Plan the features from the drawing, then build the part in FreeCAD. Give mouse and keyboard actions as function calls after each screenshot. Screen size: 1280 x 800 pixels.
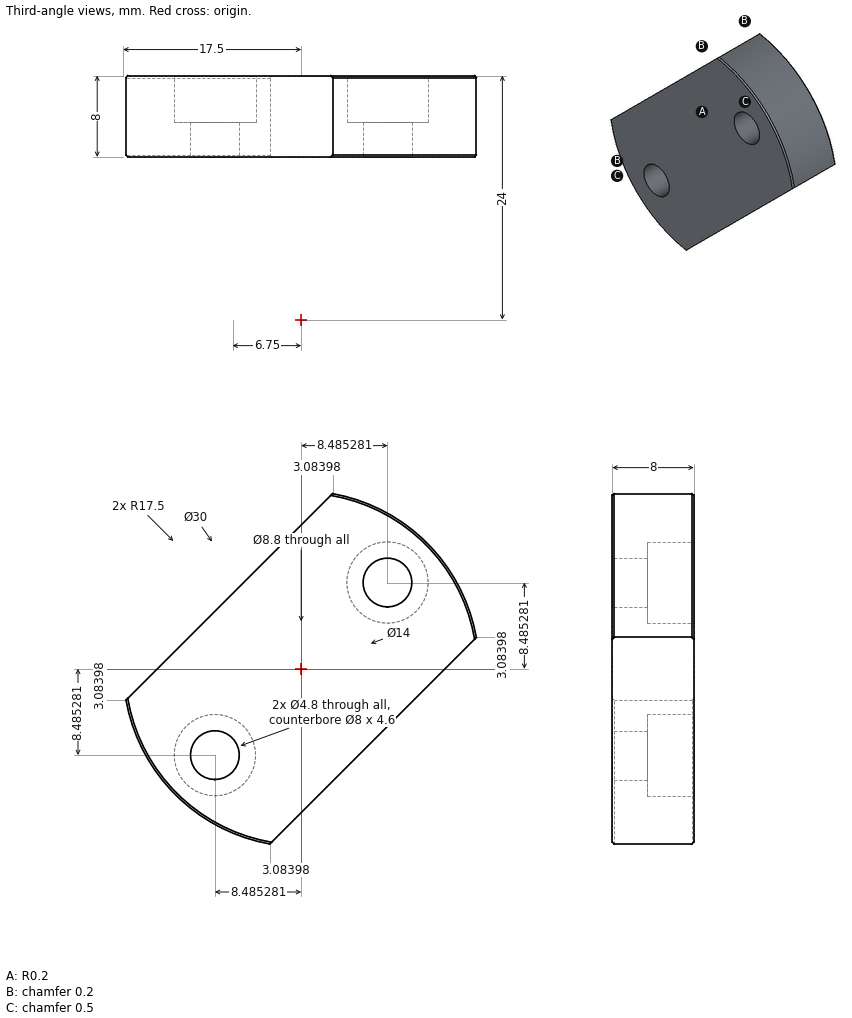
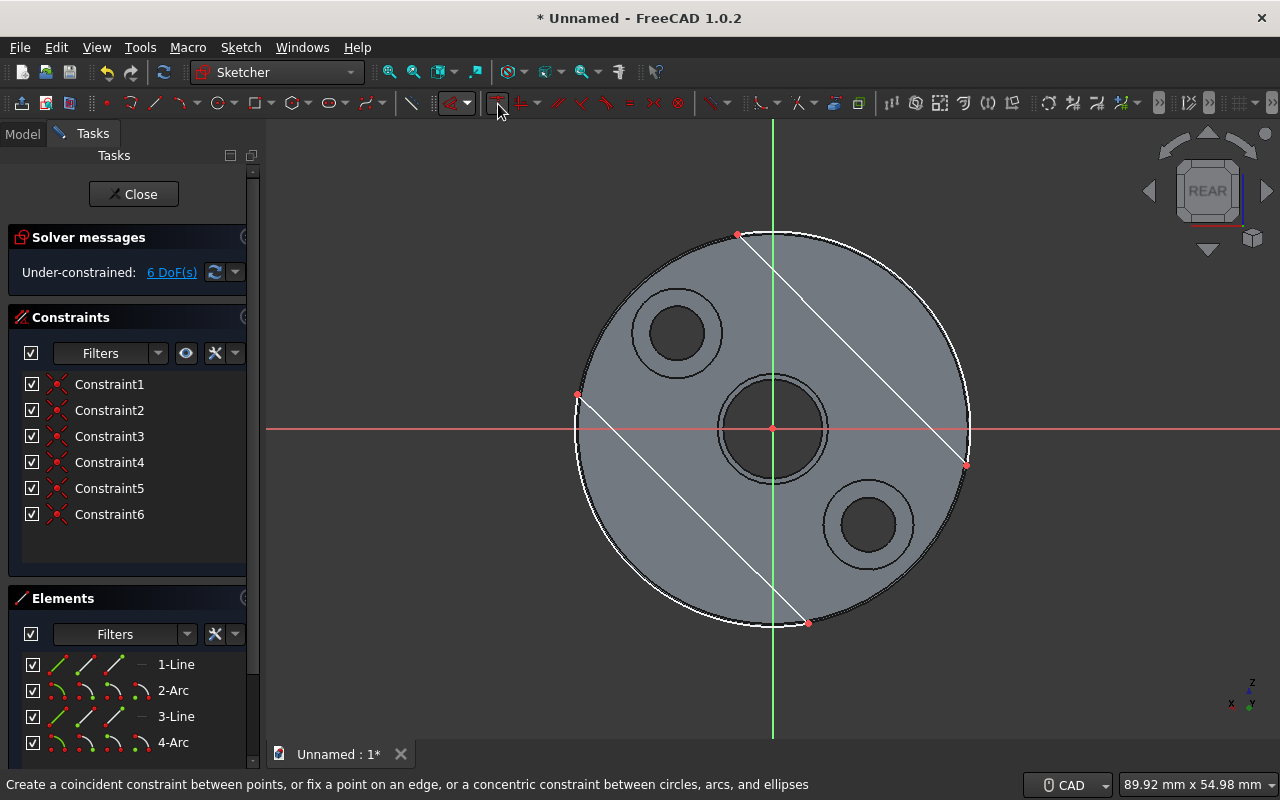
click(955, 353)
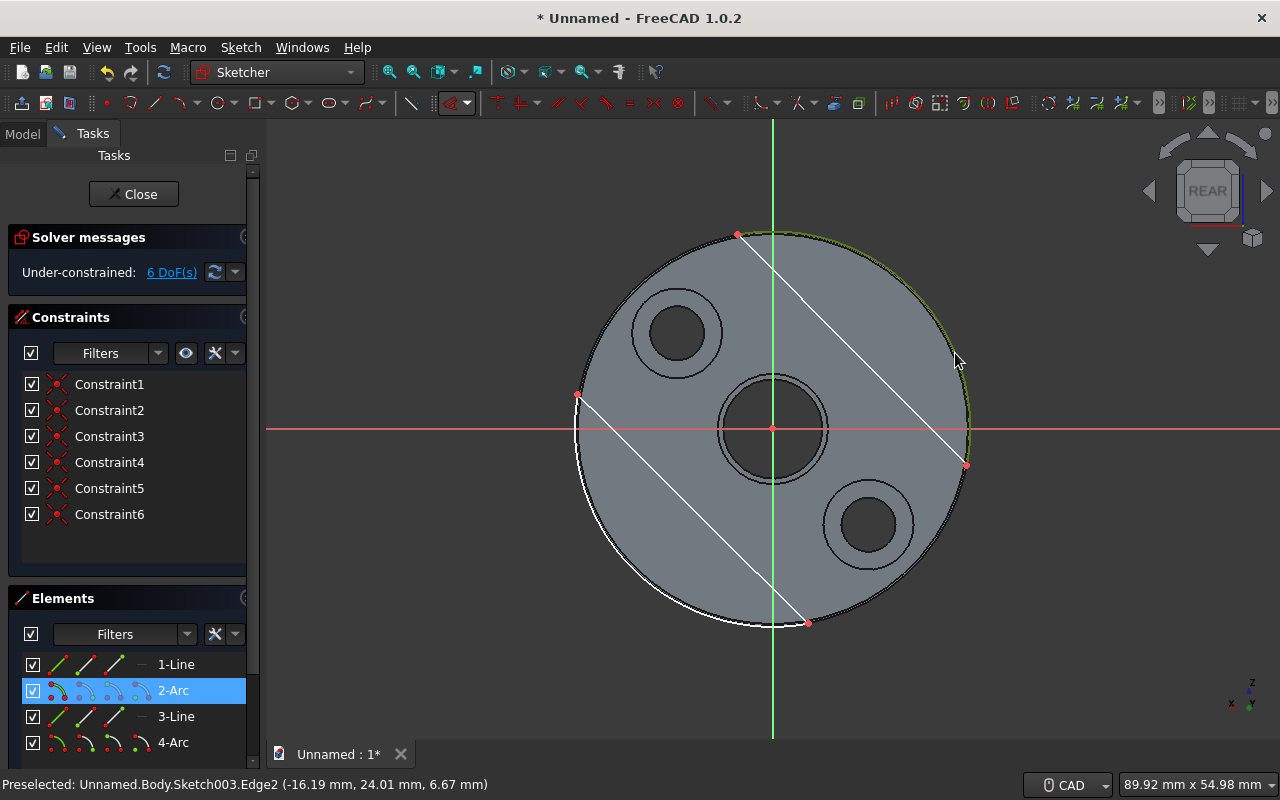
click(591, 507)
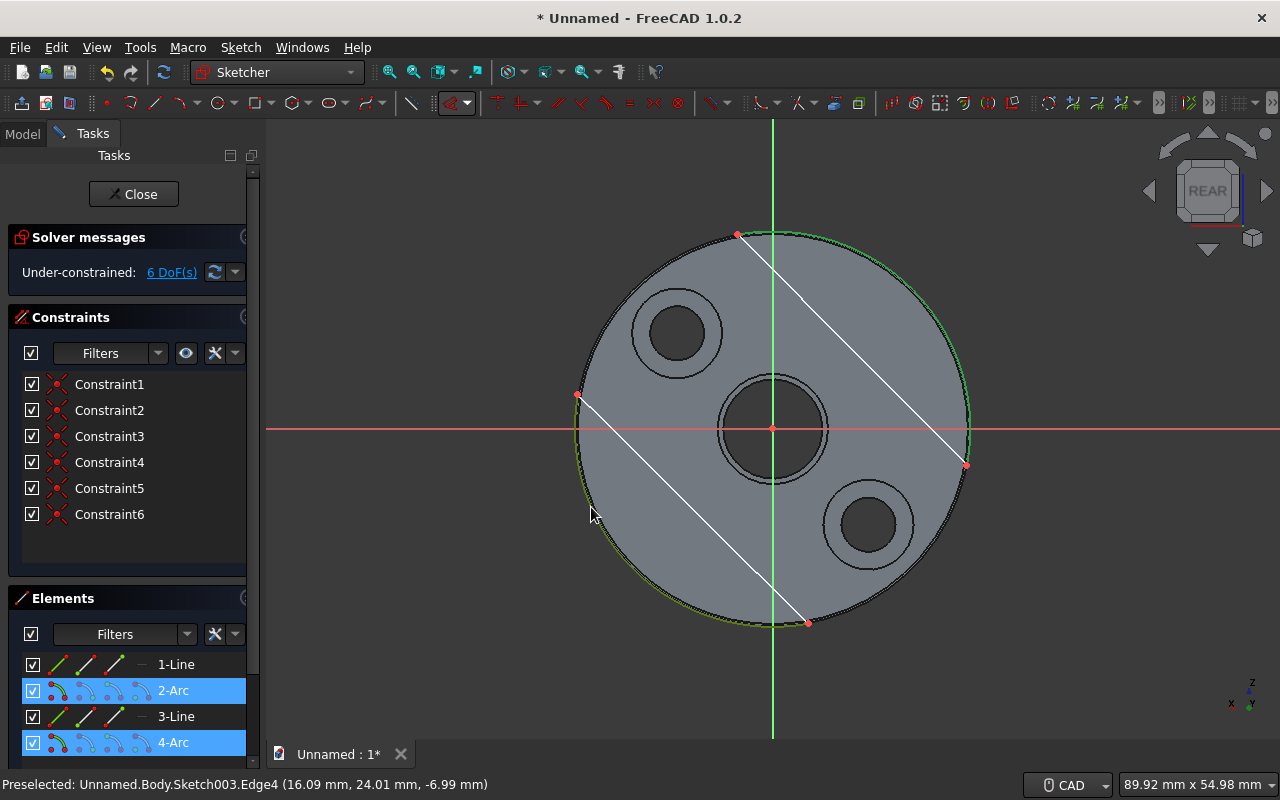
click(630, 104)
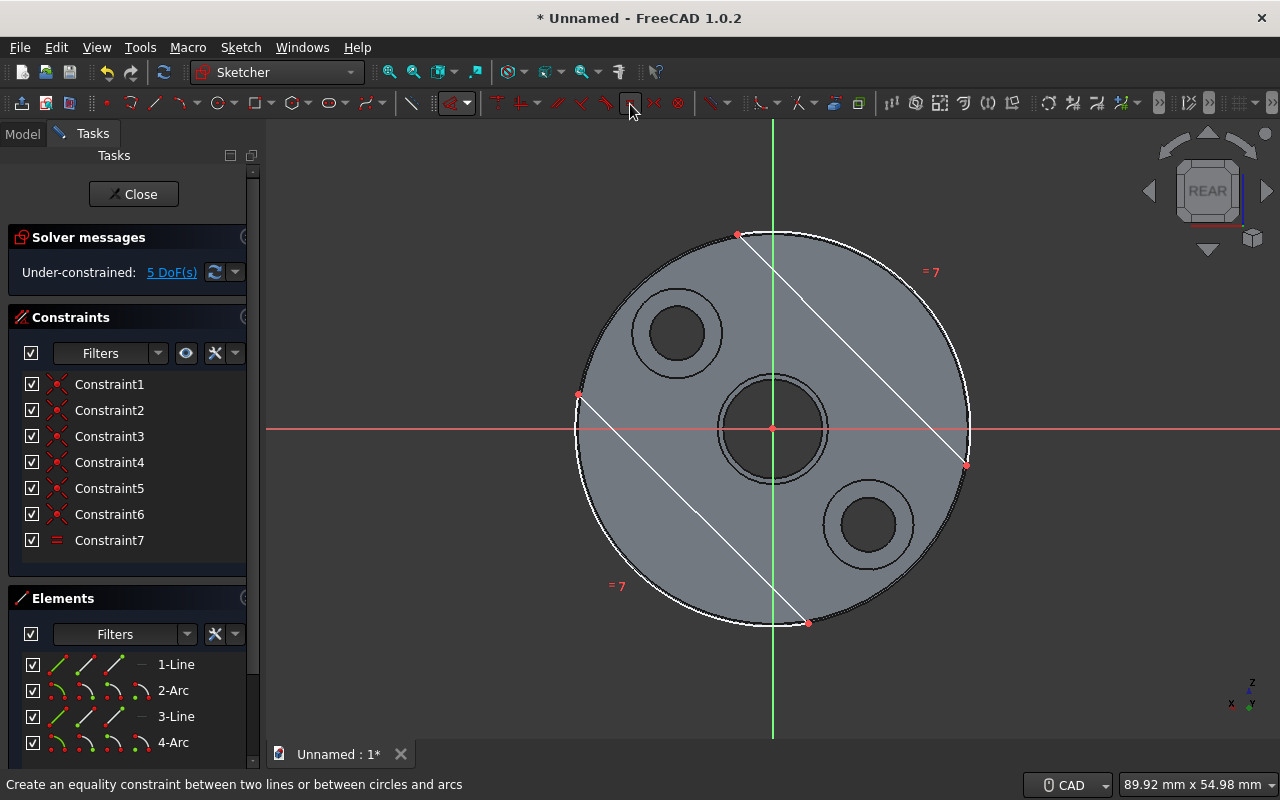
click(955, 353)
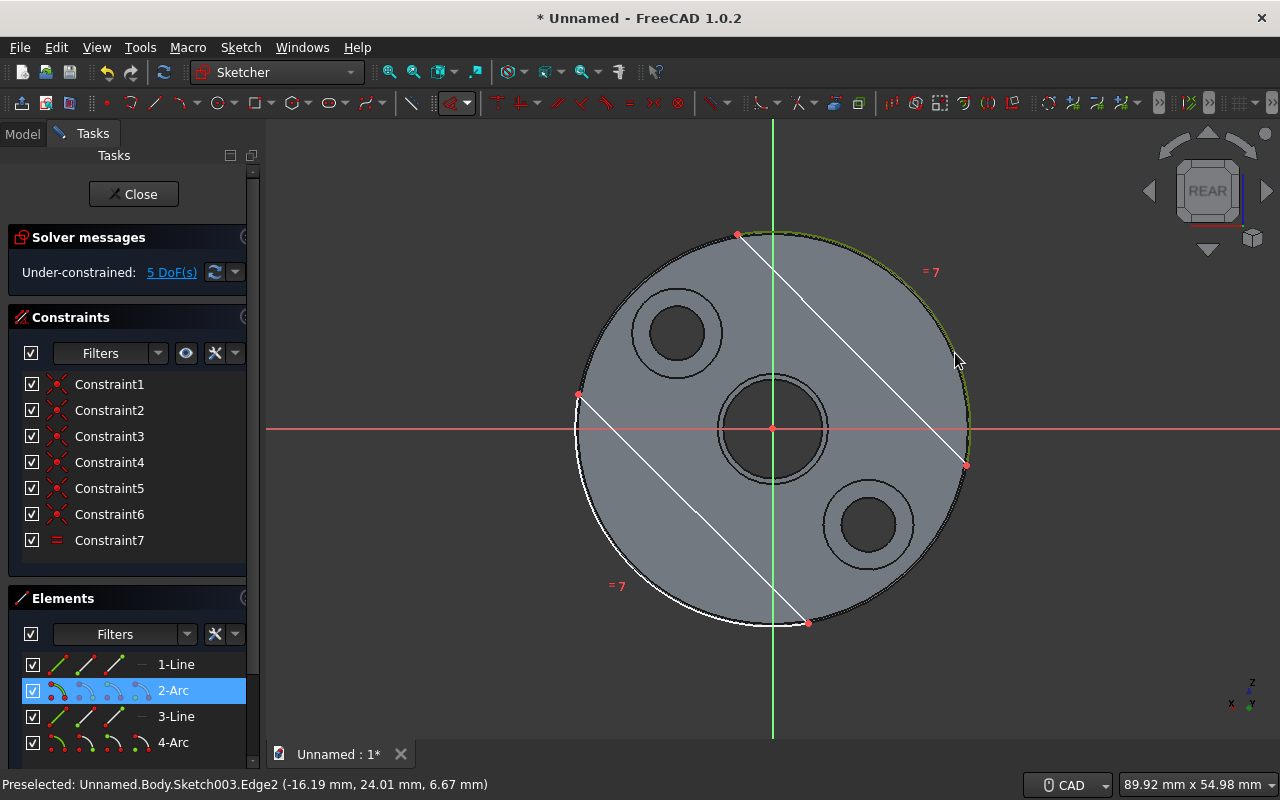
click(470, 104)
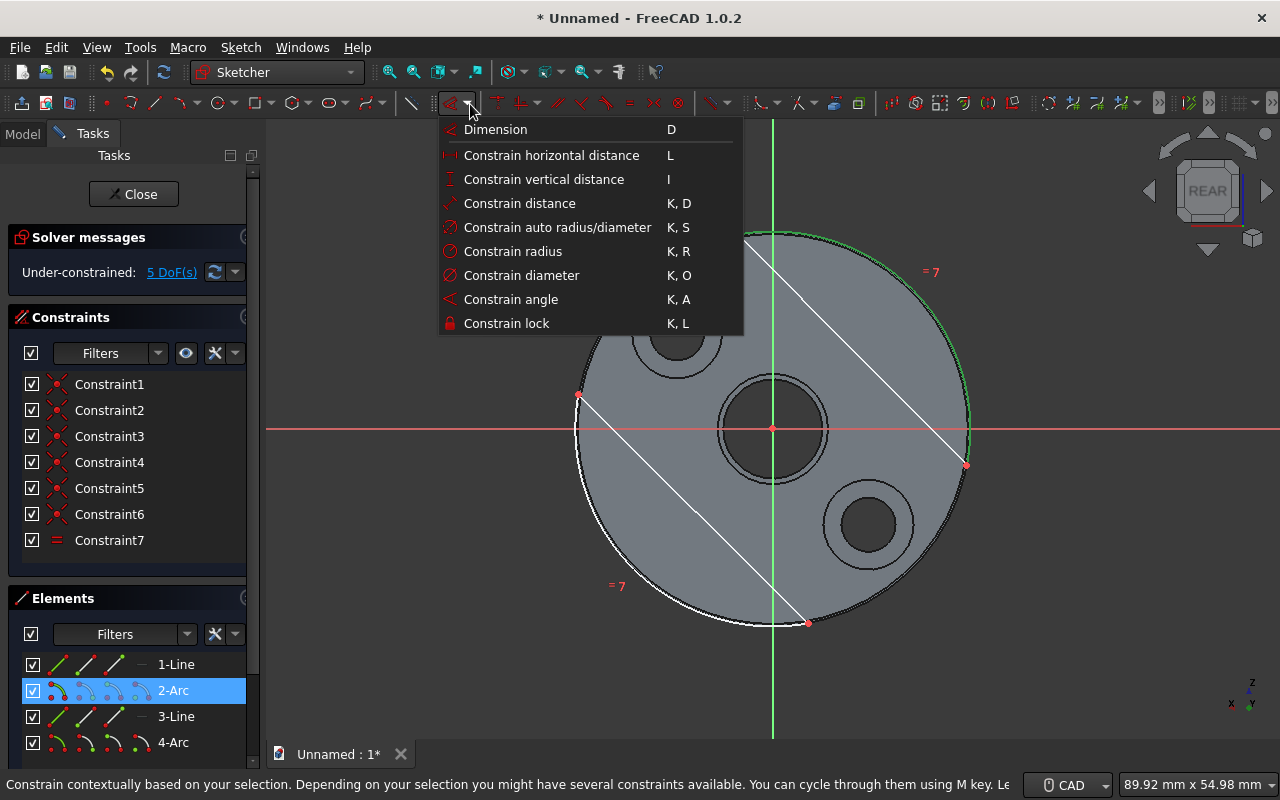
click(591, 251)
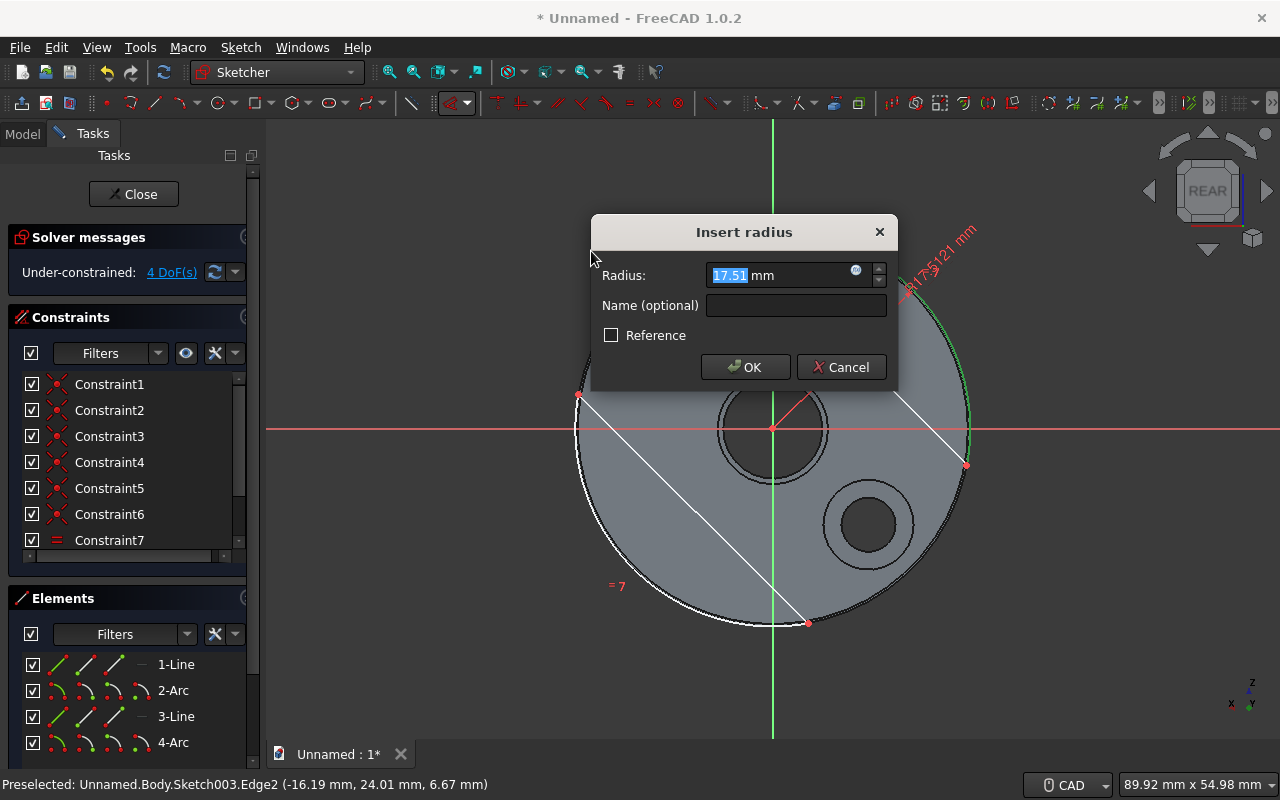
text(17.5)
key(Return)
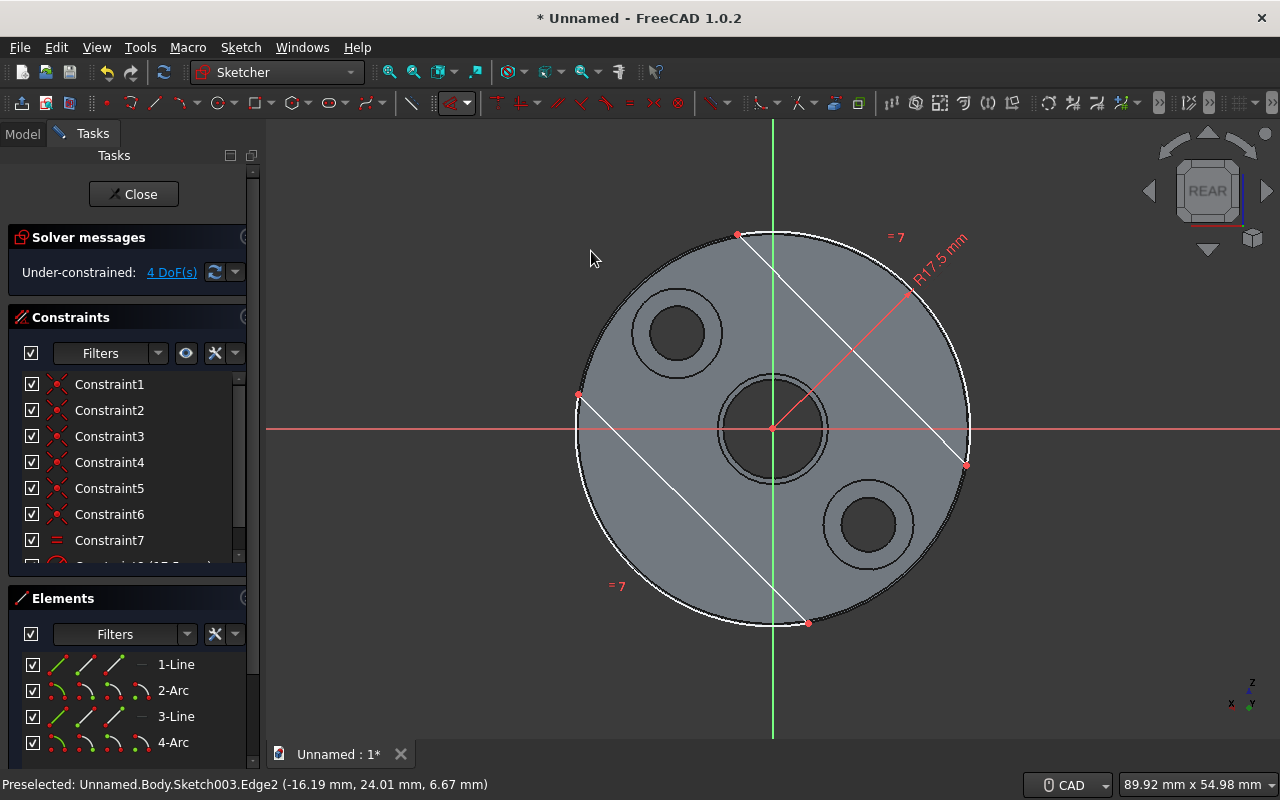
click(738, 235)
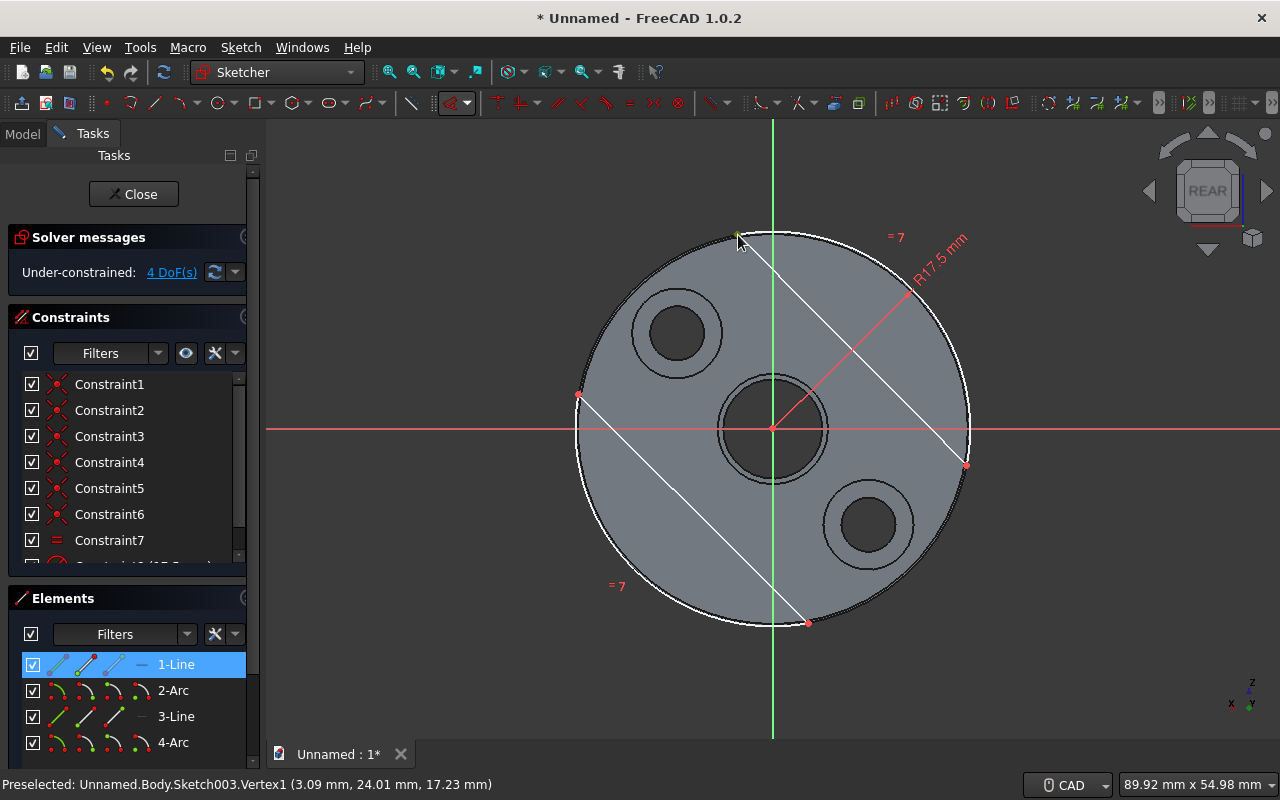
click(470, 104)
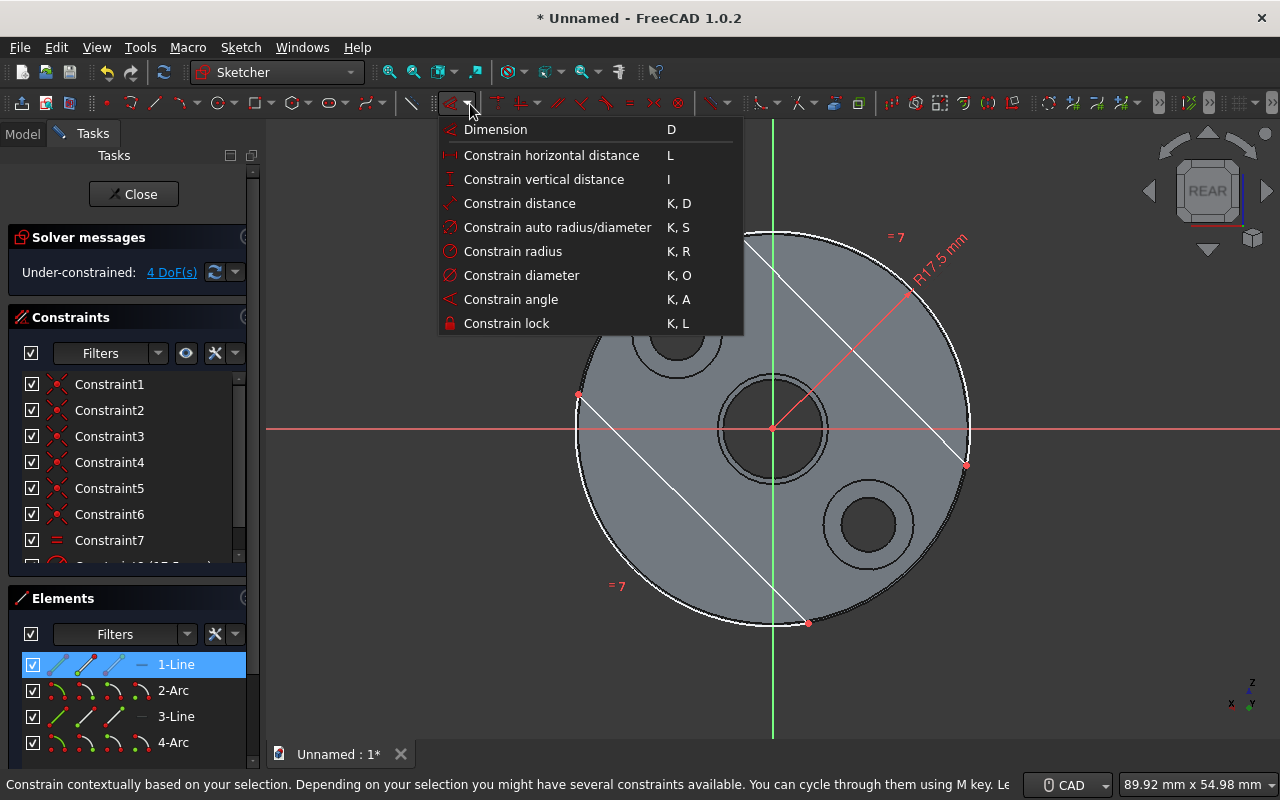
click(591, 155)